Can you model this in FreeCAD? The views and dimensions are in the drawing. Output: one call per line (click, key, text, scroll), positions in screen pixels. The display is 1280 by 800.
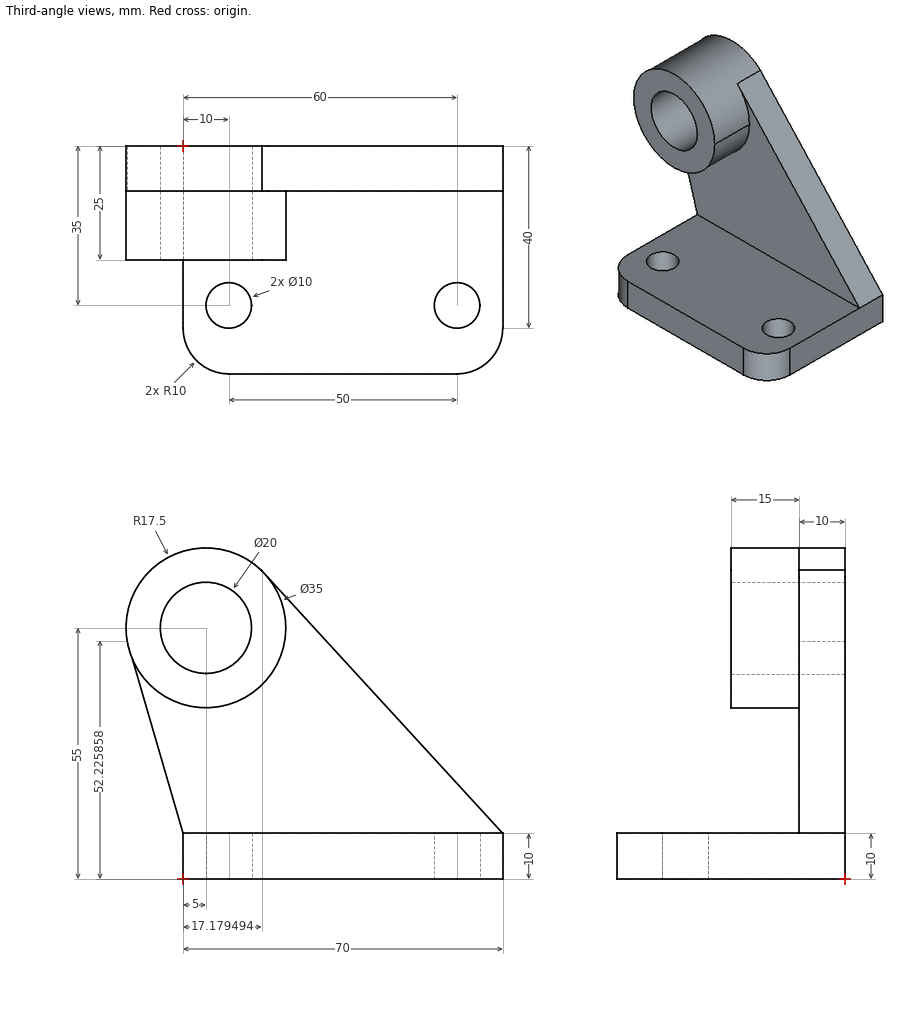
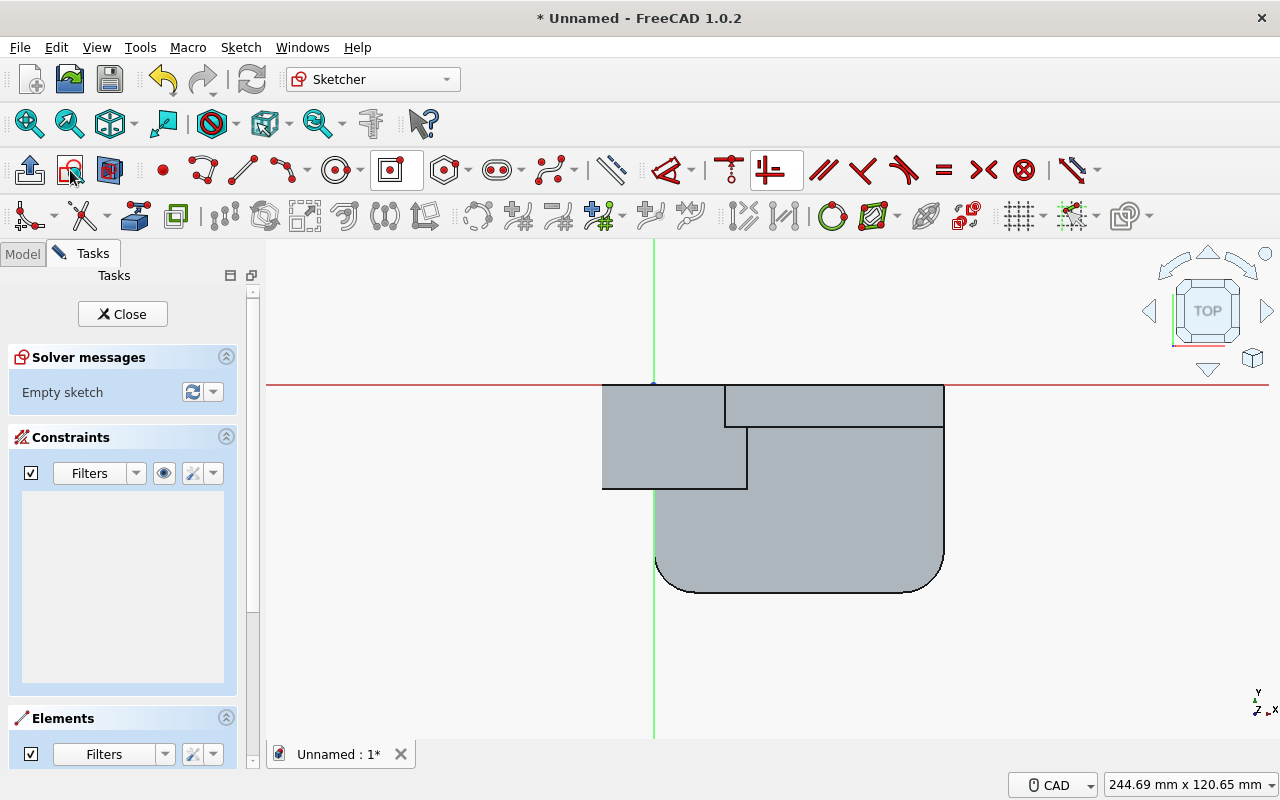
scroll(891, 443, up, 3)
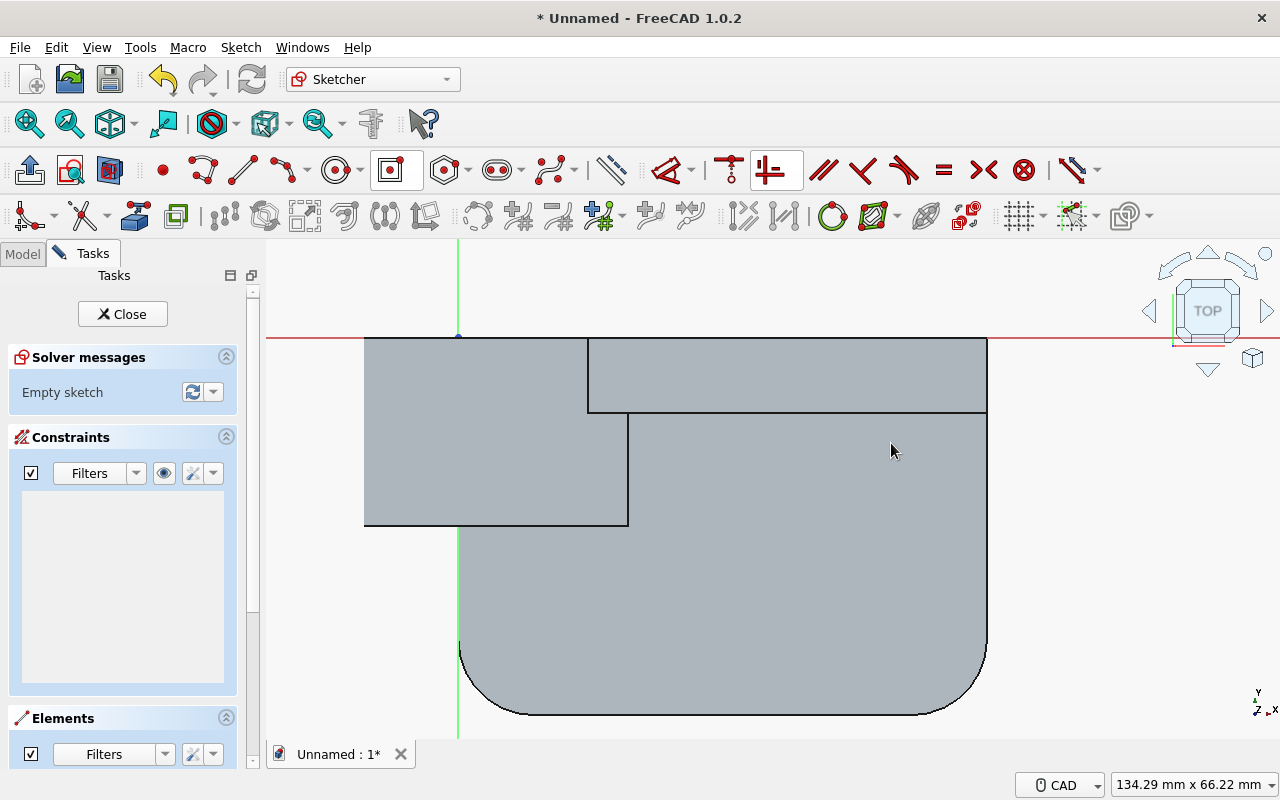
click(336, 170)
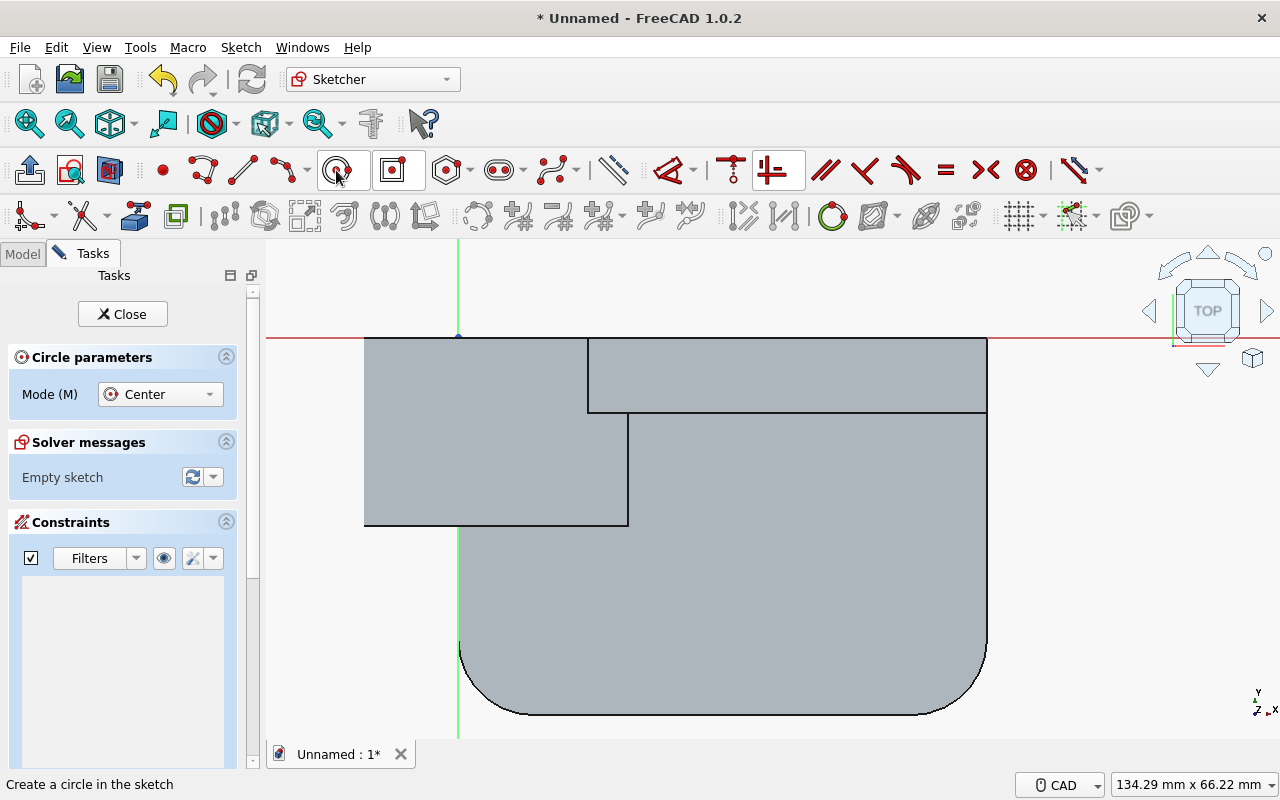
click(534, 602)
click(561, 575)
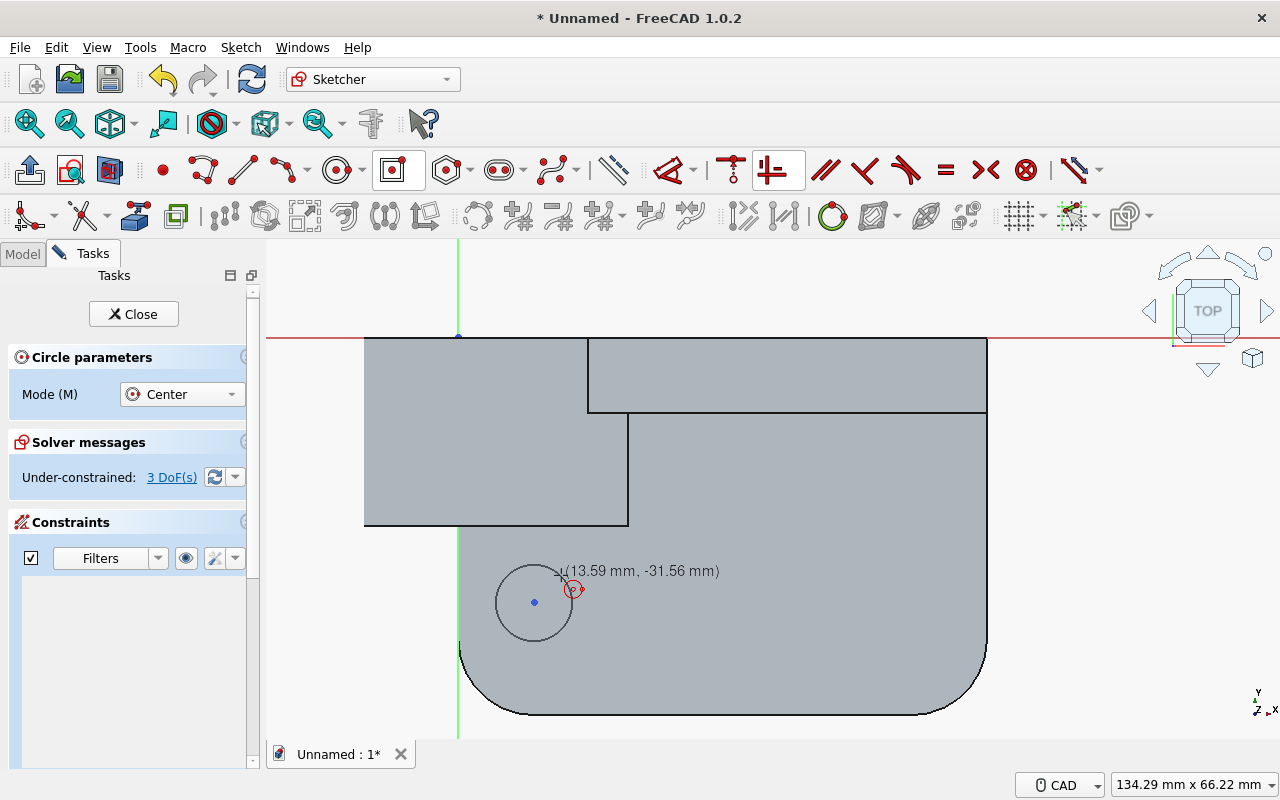
click(911, 602)
click(938, 575)
key(Escape)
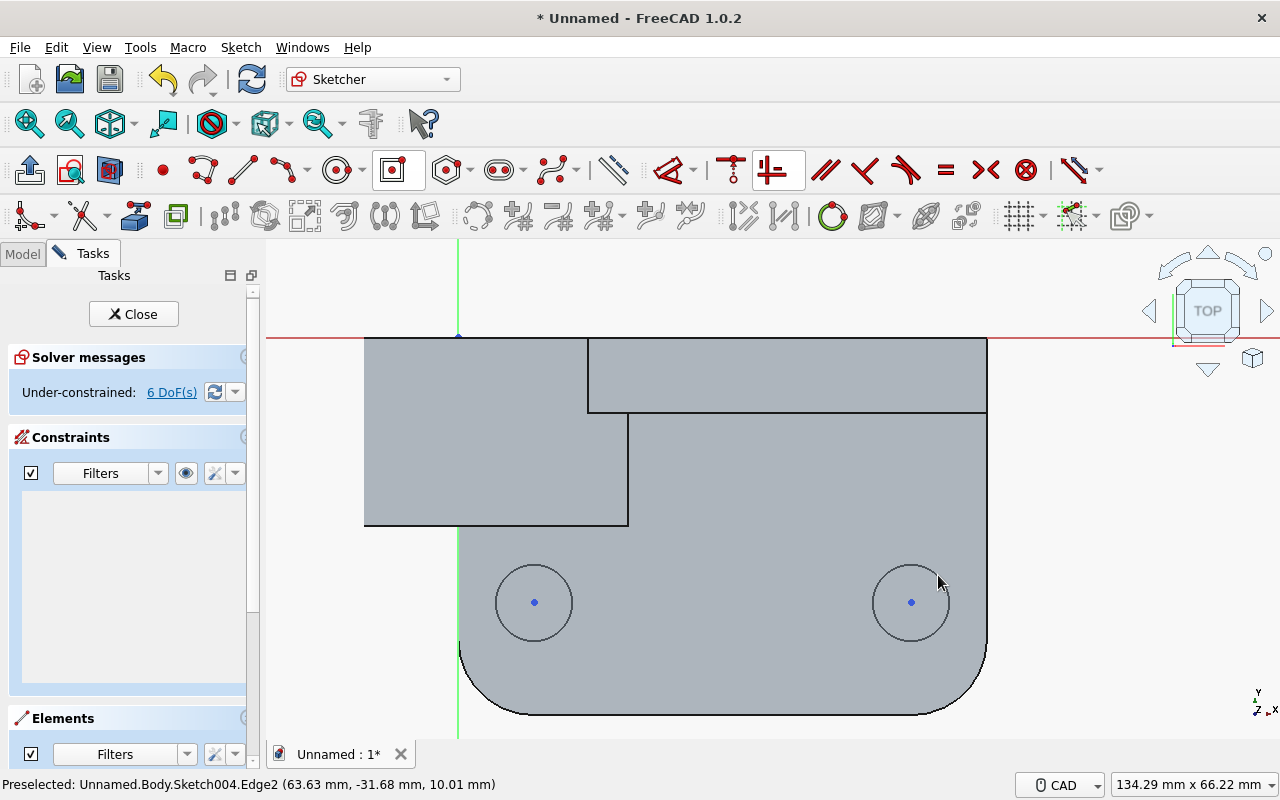
click(561, 576)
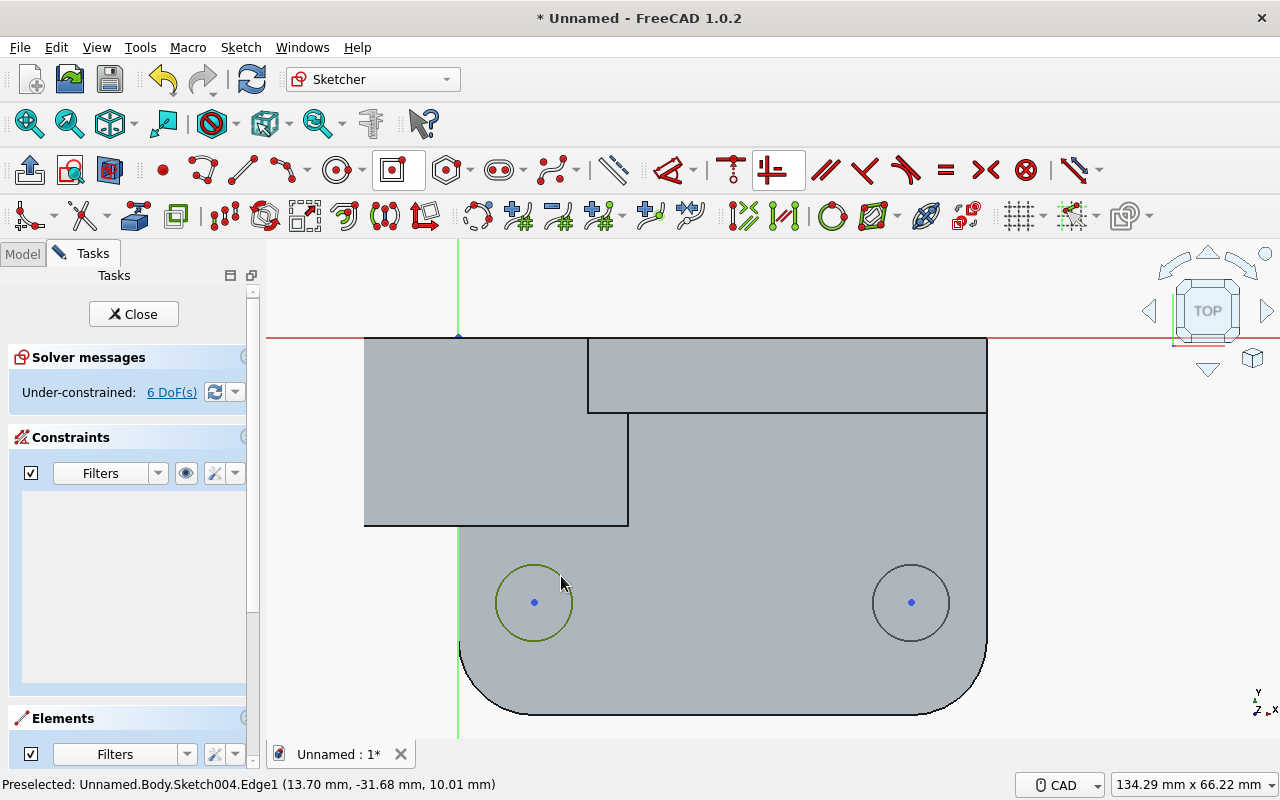
click(938, 576)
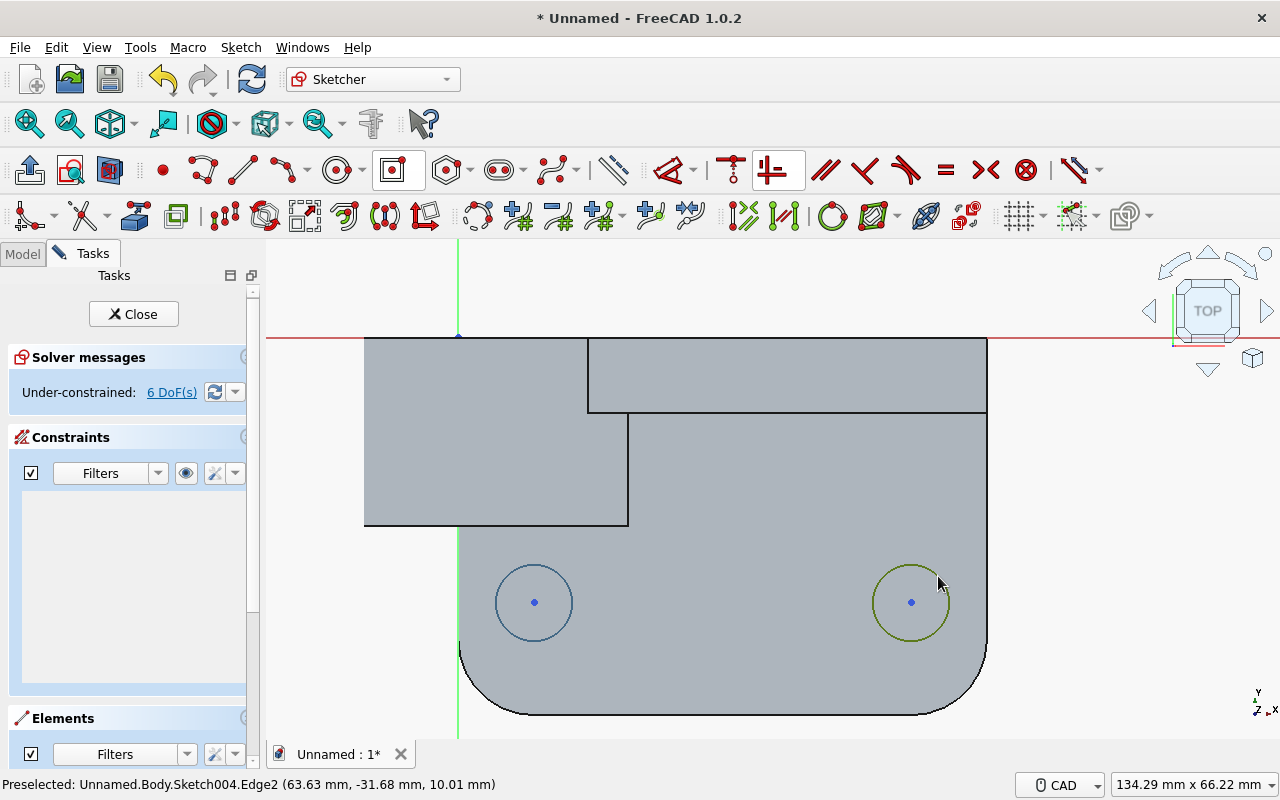
click(946, 170)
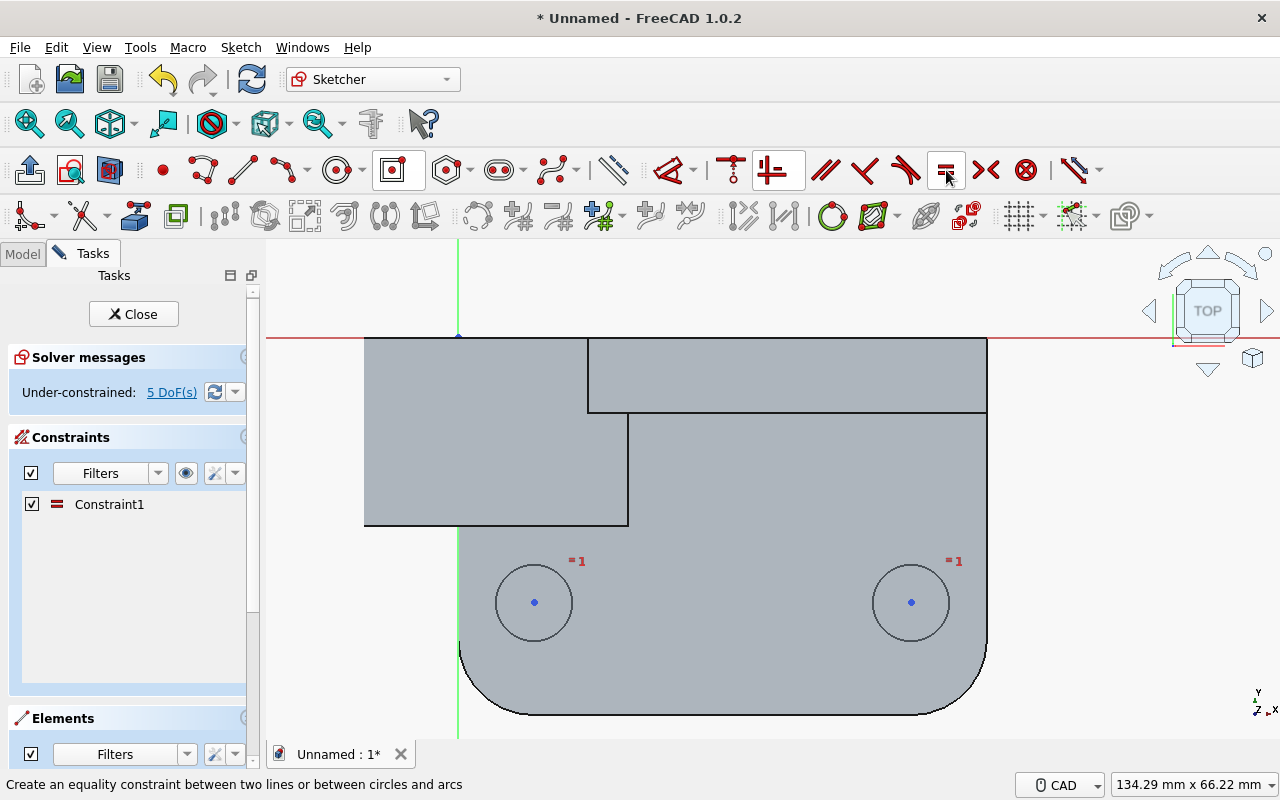
key(d)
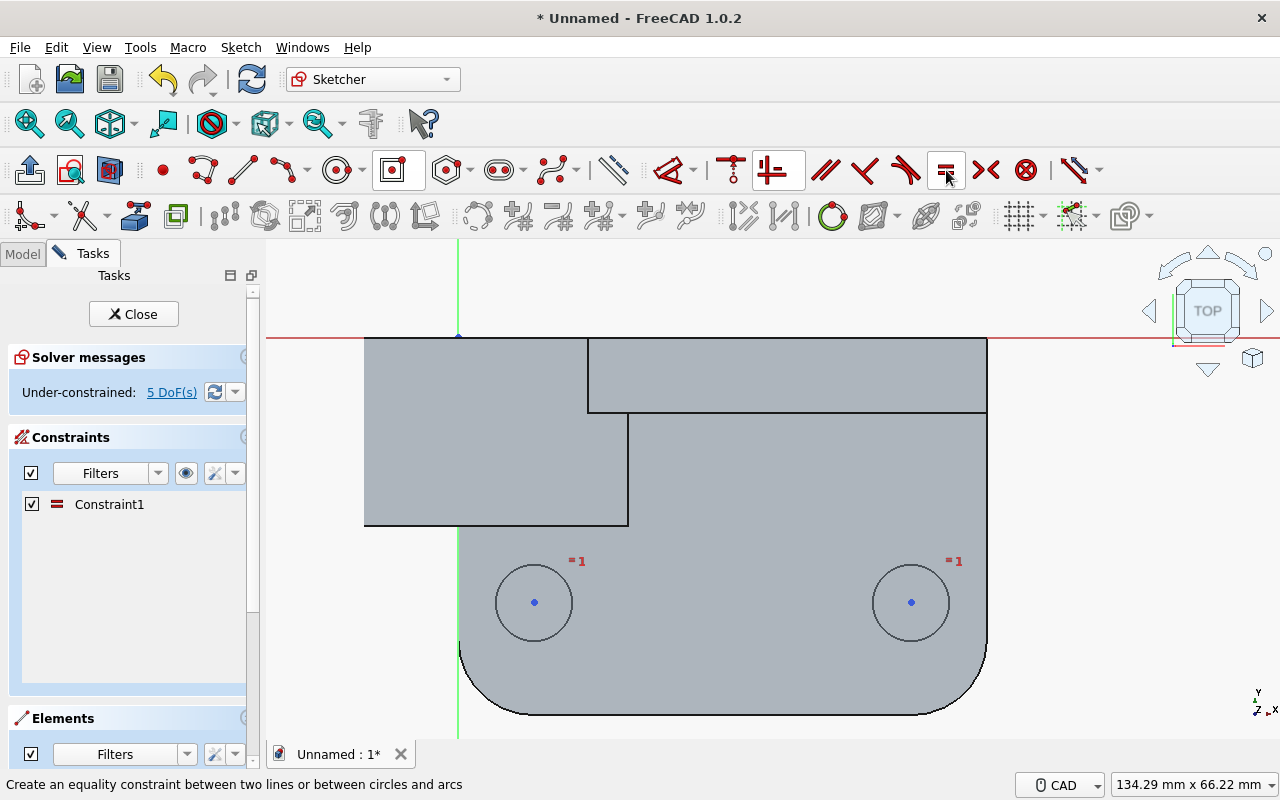
click(561, 576)
click(584, 553)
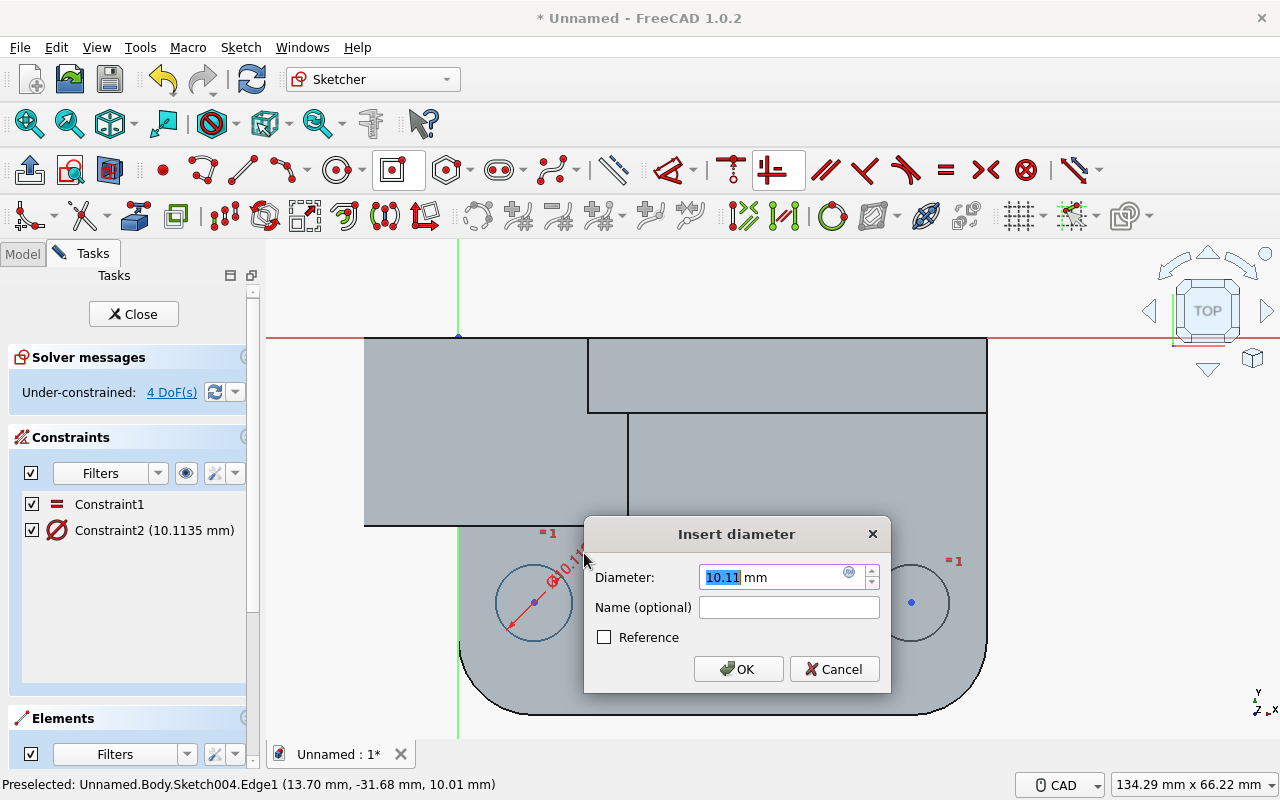
text(10)
key(Return)